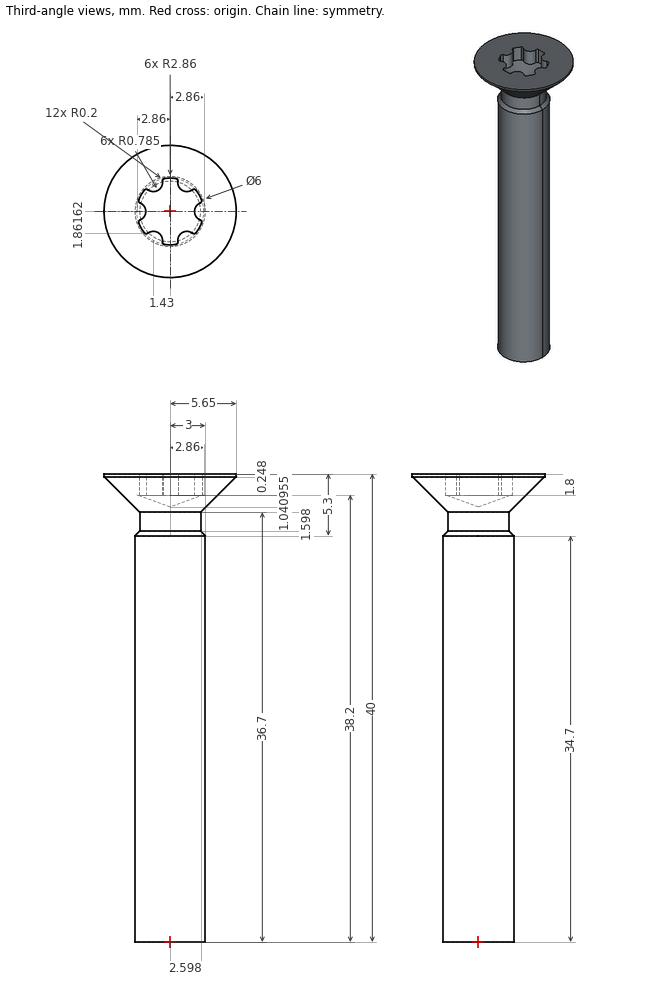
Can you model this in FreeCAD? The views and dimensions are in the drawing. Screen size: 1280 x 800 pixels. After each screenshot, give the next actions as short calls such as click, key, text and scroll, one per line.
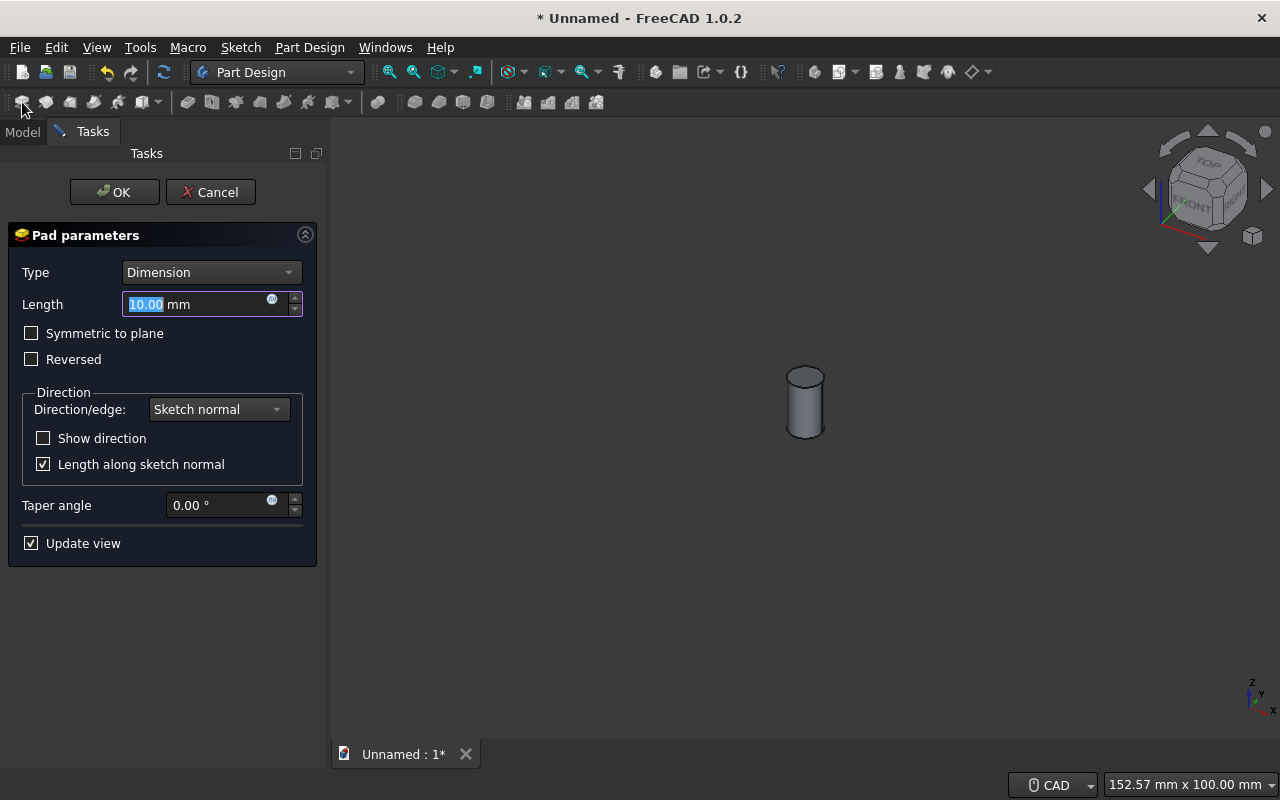
text(34.7)
key(Tab)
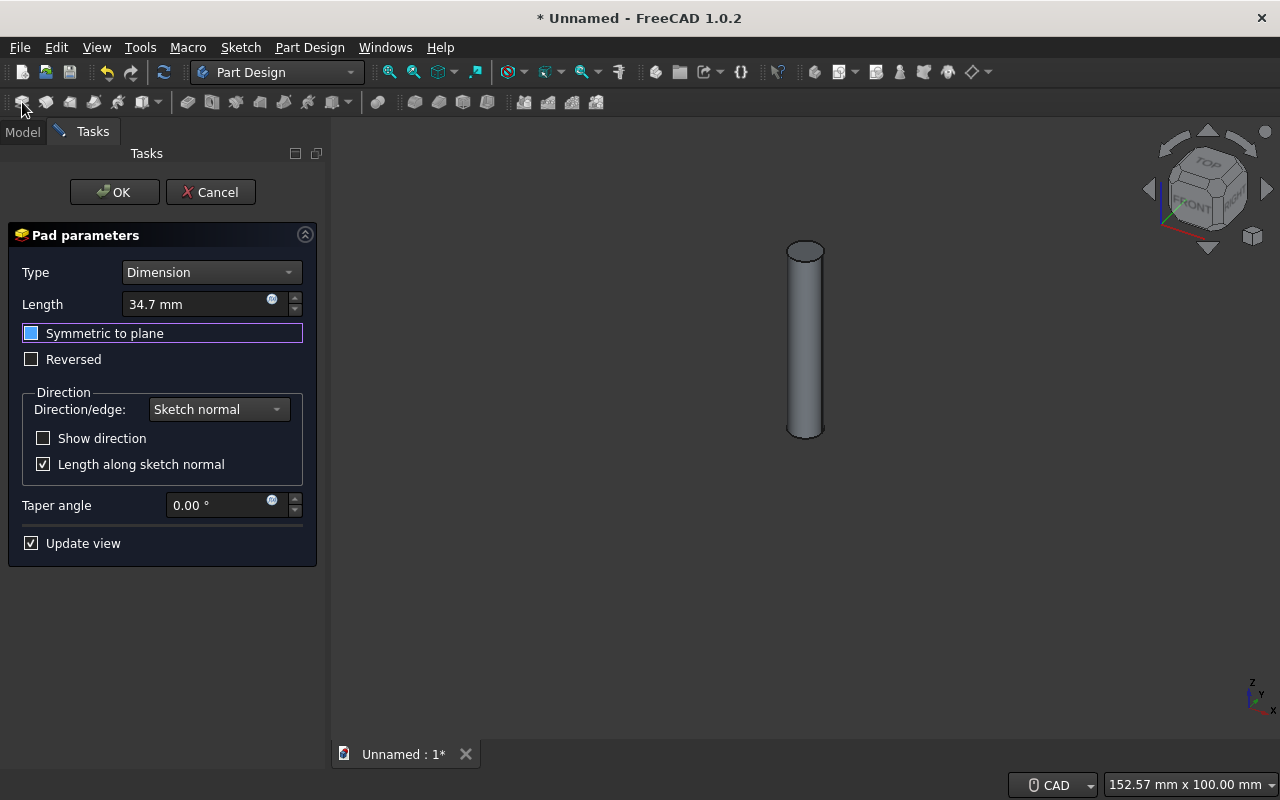
click(115, 192)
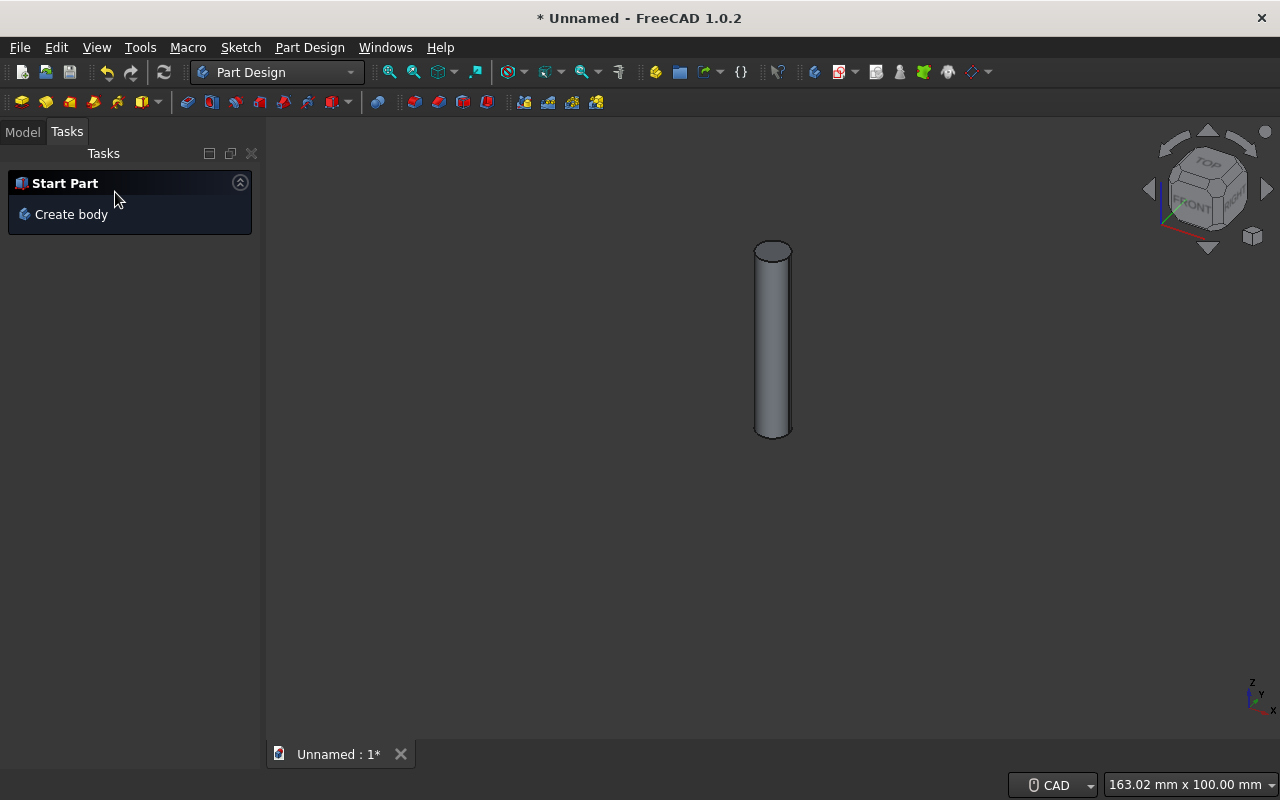
key(v)
key(f)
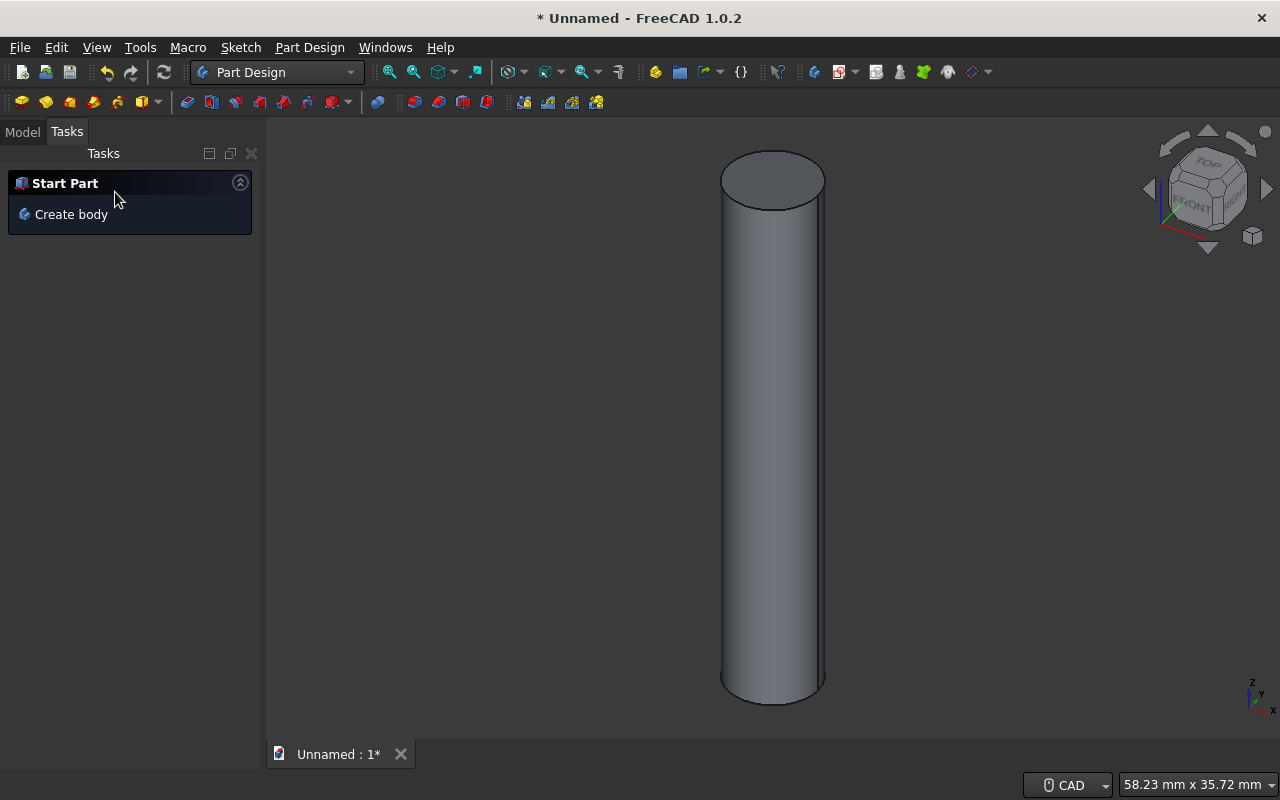
click(840, 72)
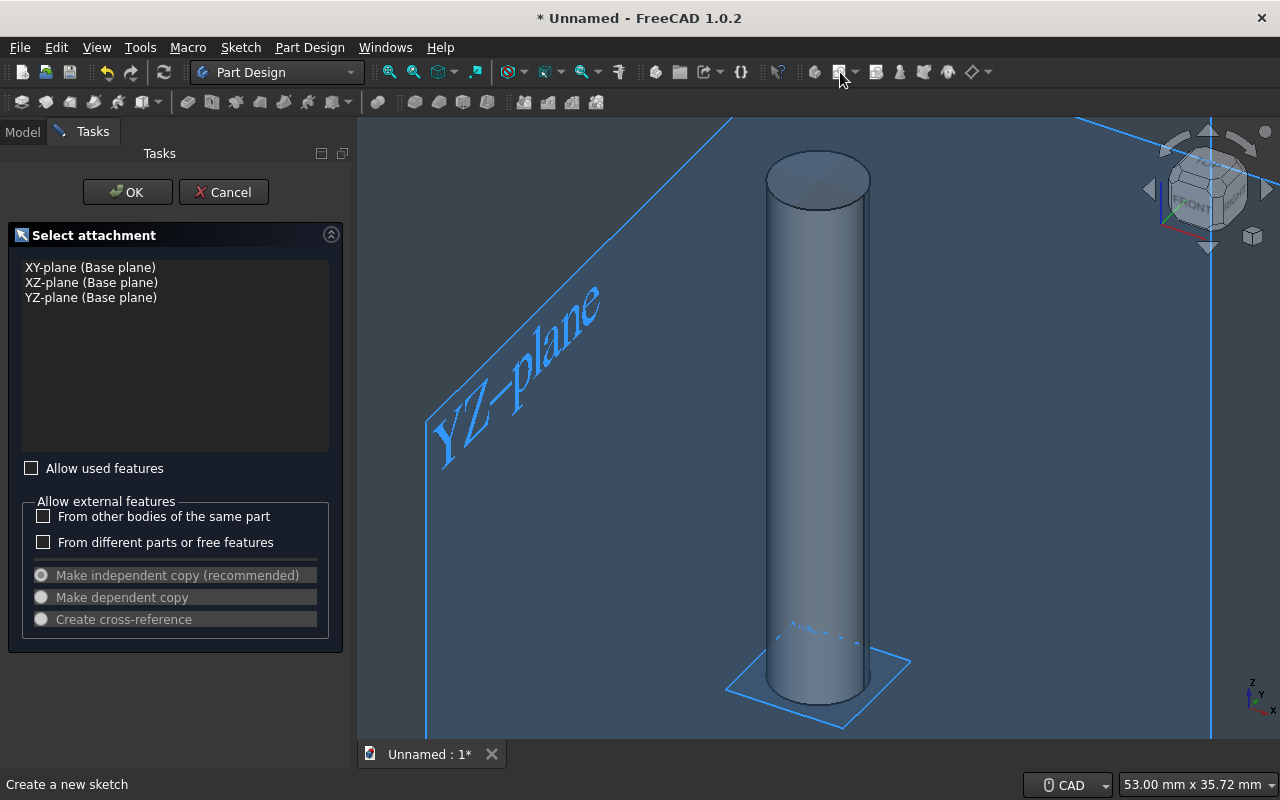
click(82, 282)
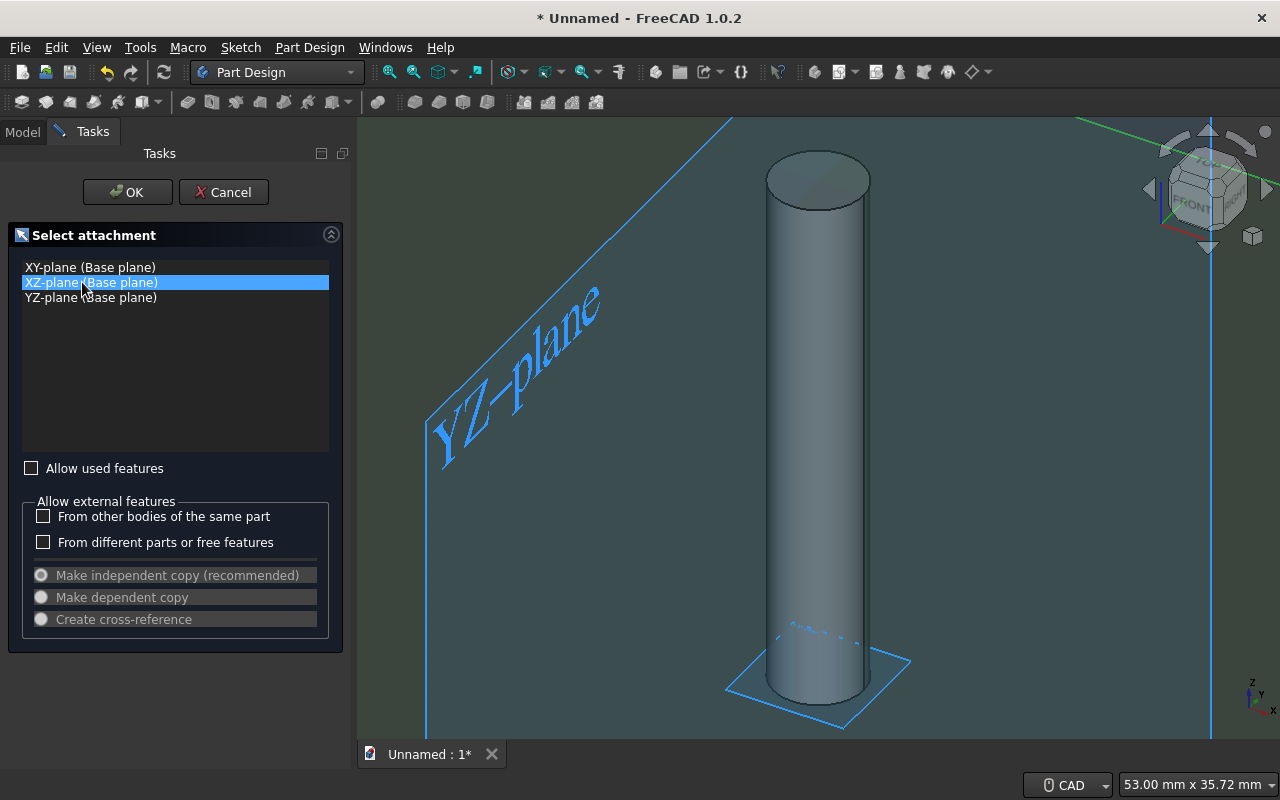
click(128, 192)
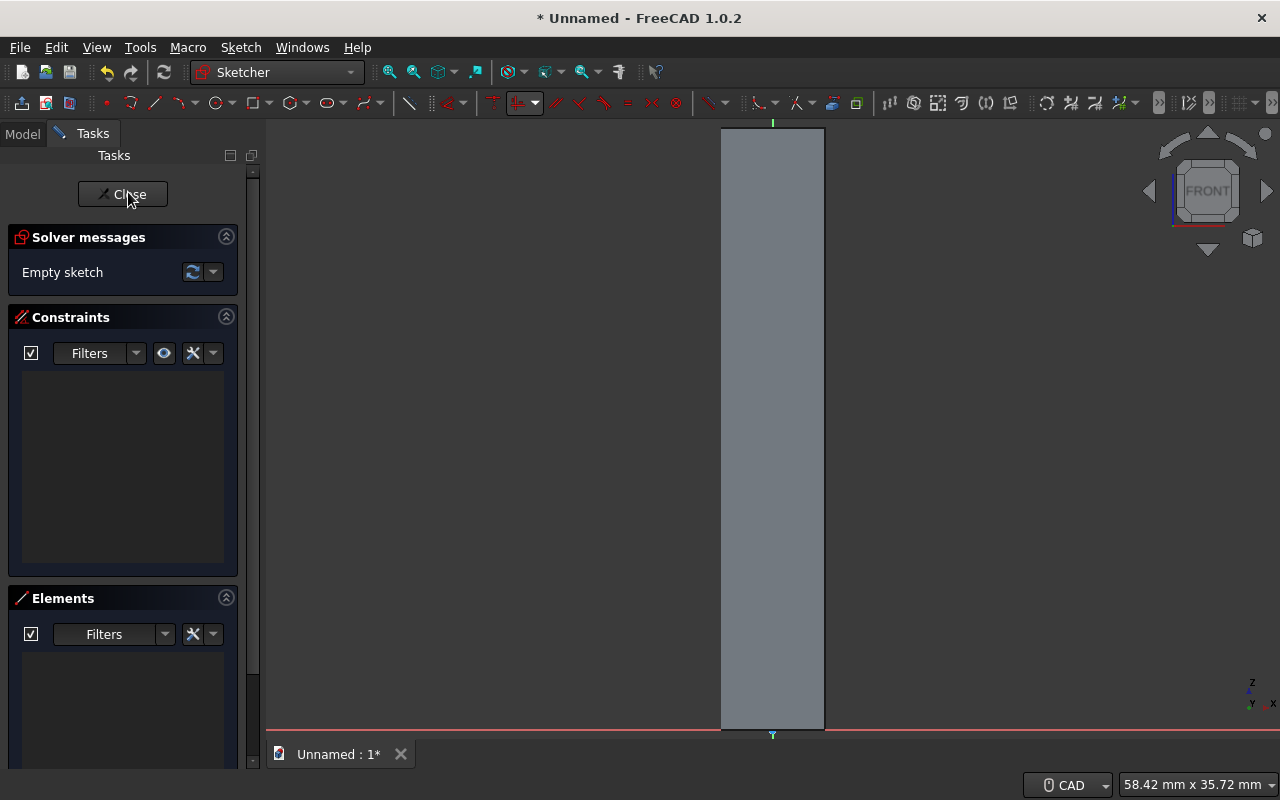
key(q)
key(s)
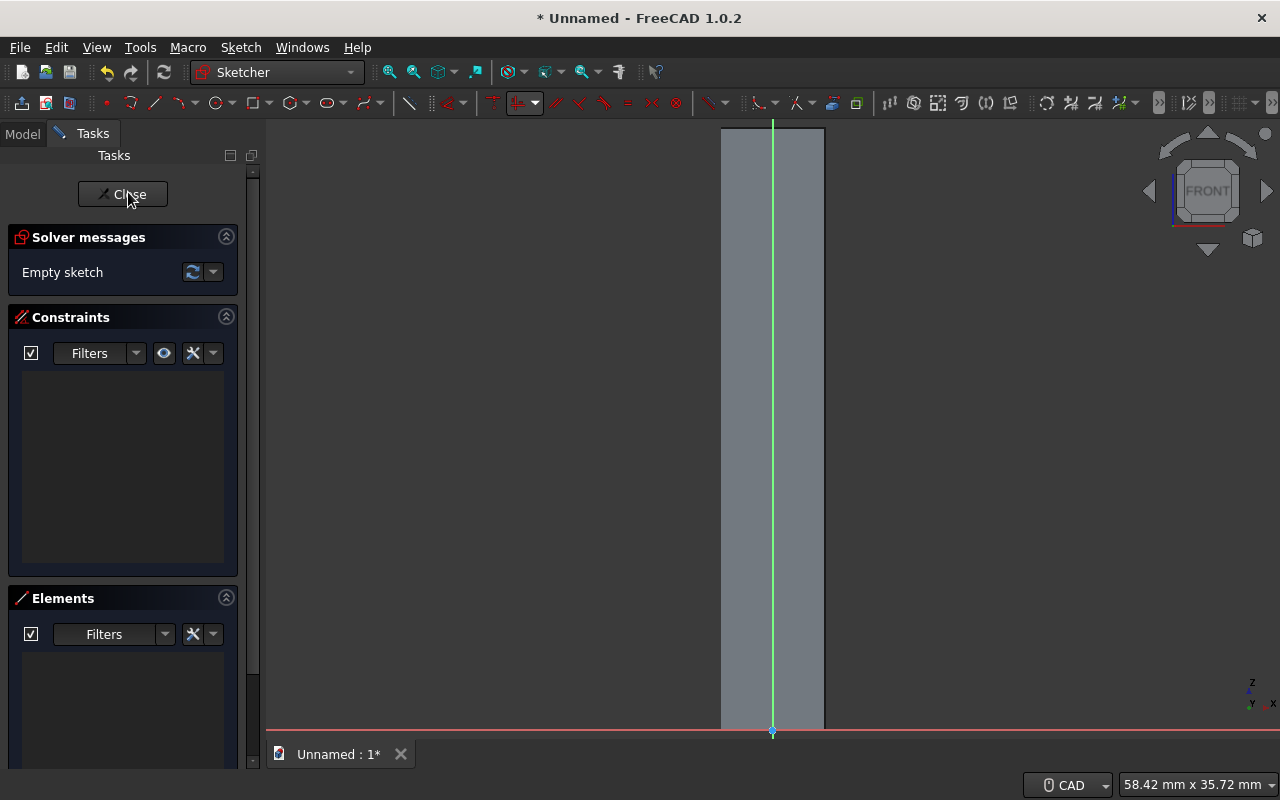
scroll(704, 429, down, 5)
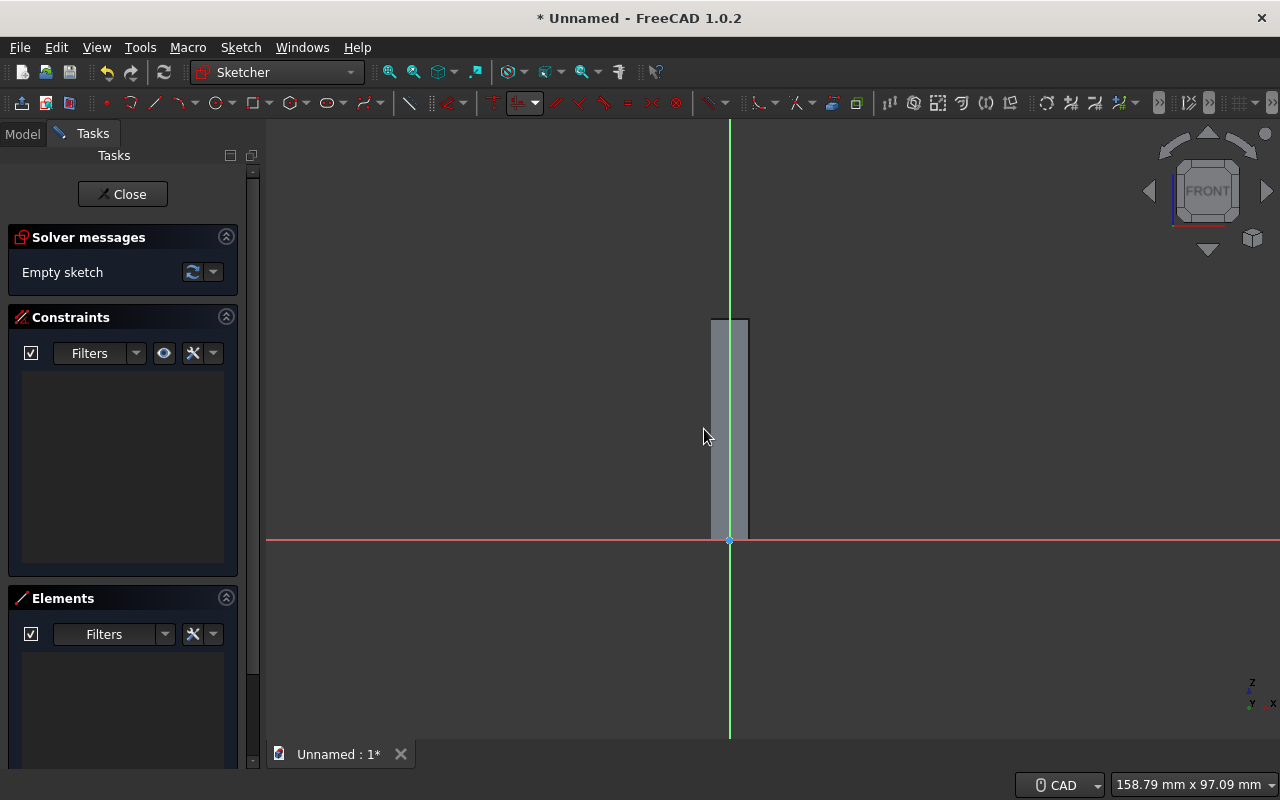
scroll(752, 289, up, 12)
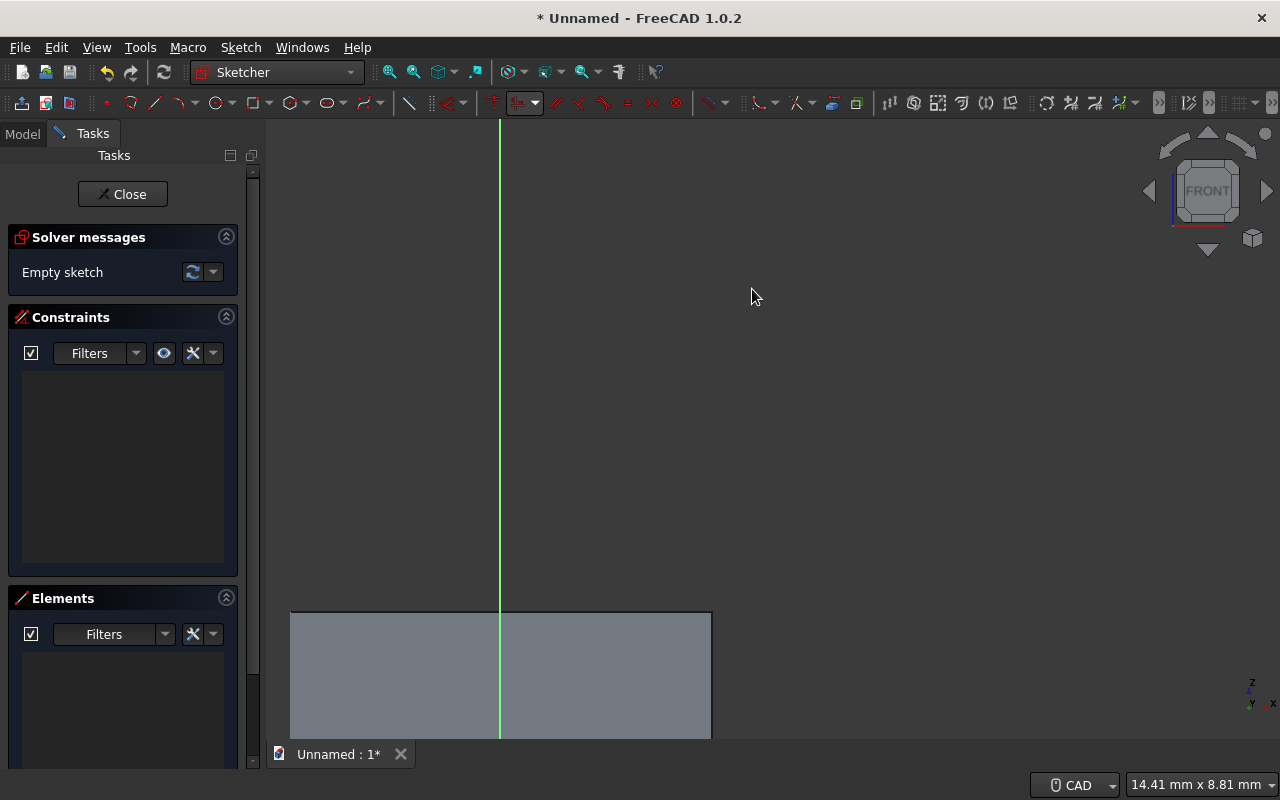
click(132, 104)